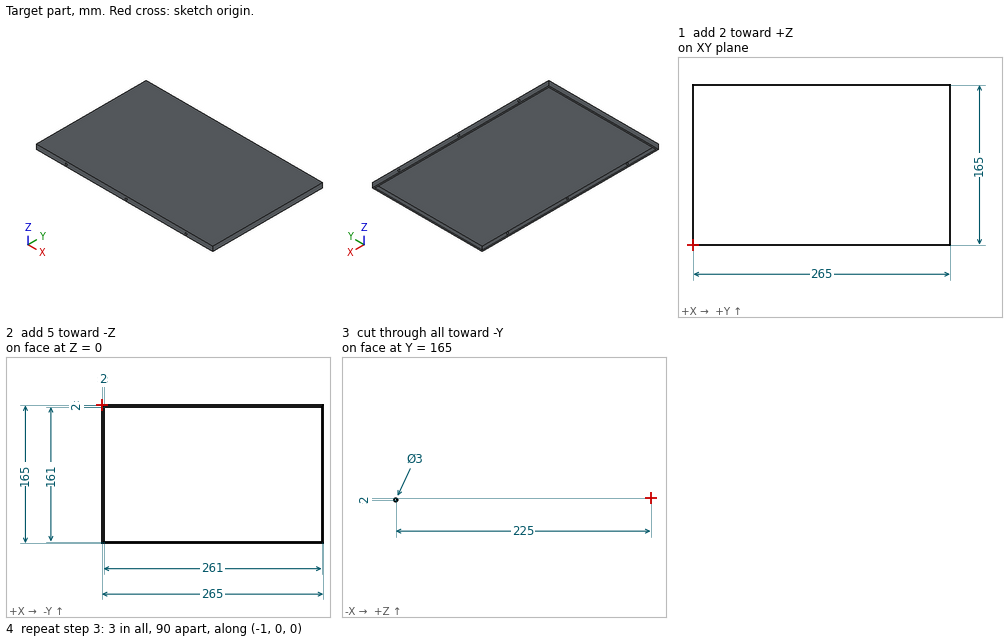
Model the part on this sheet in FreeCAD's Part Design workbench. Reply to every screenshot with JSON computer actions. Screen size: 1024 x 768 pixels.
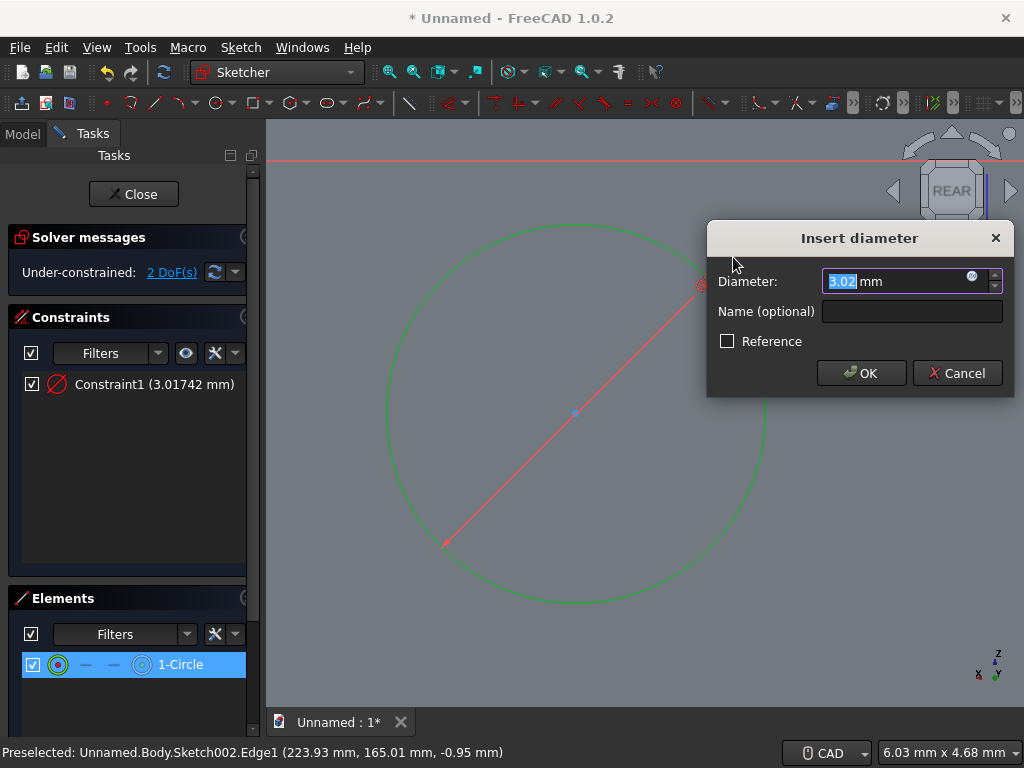
{"action": "type", "text": "3"}
{"action": "key", "text": "Return"}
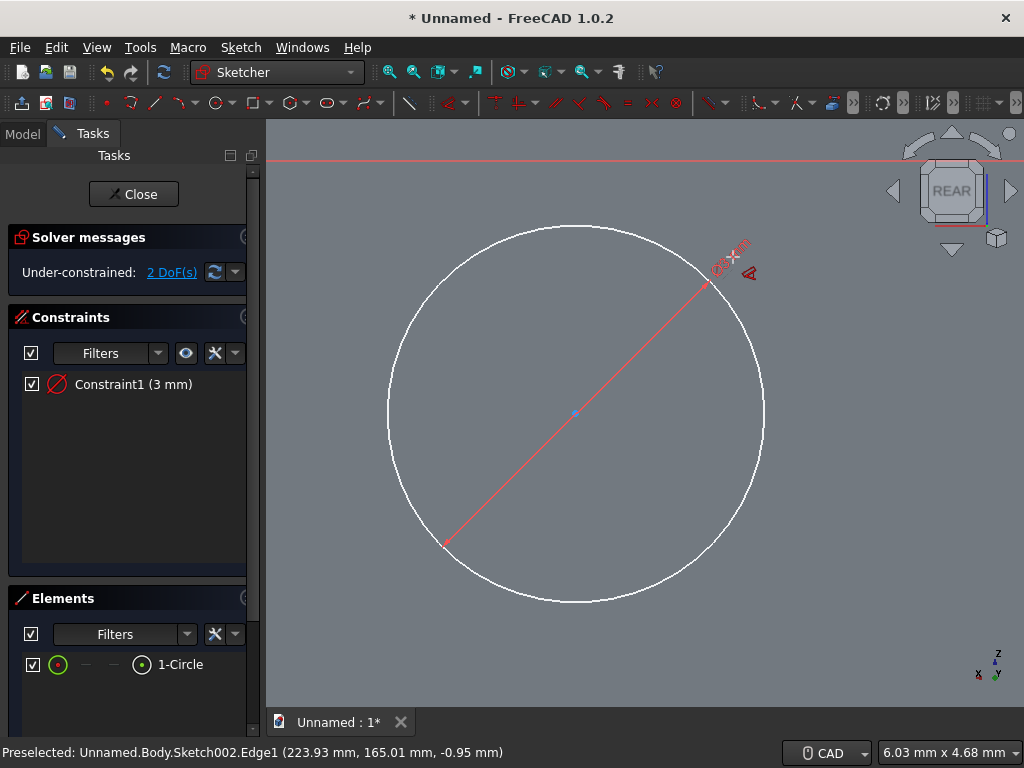
{"action": "left_click", "coordinate": [576, 414]}
{"action": "left_click", "coordinate": [542, 288]}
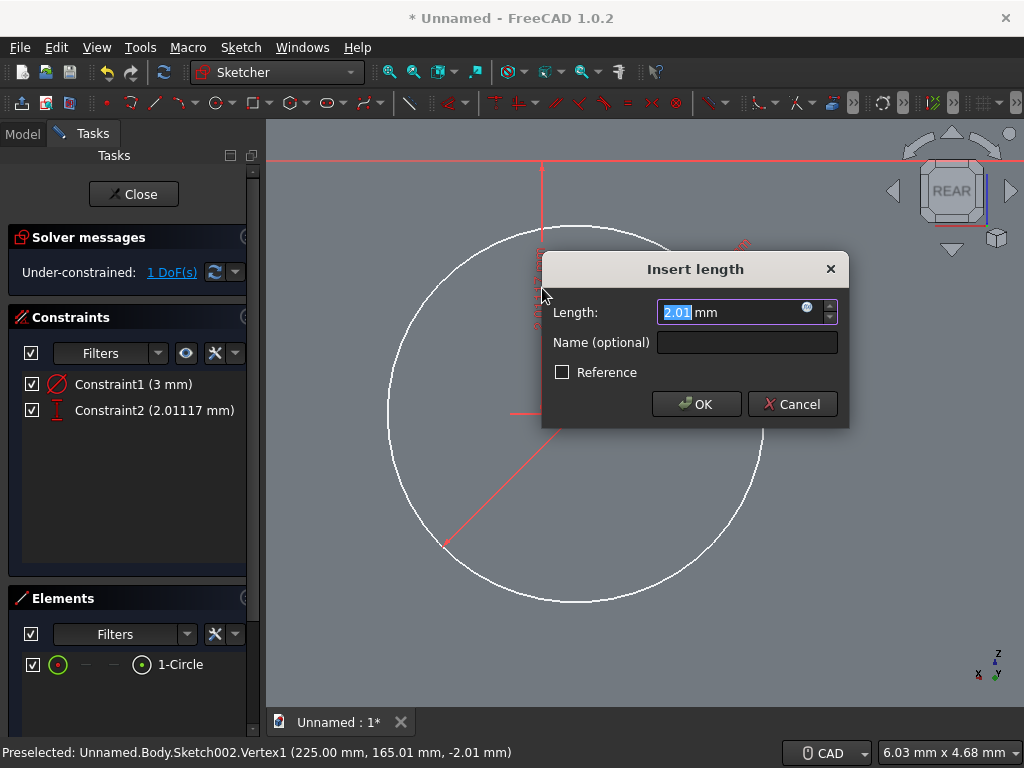
{"action": "type", "text": "2"}
{"action": "key", "text": "Return"}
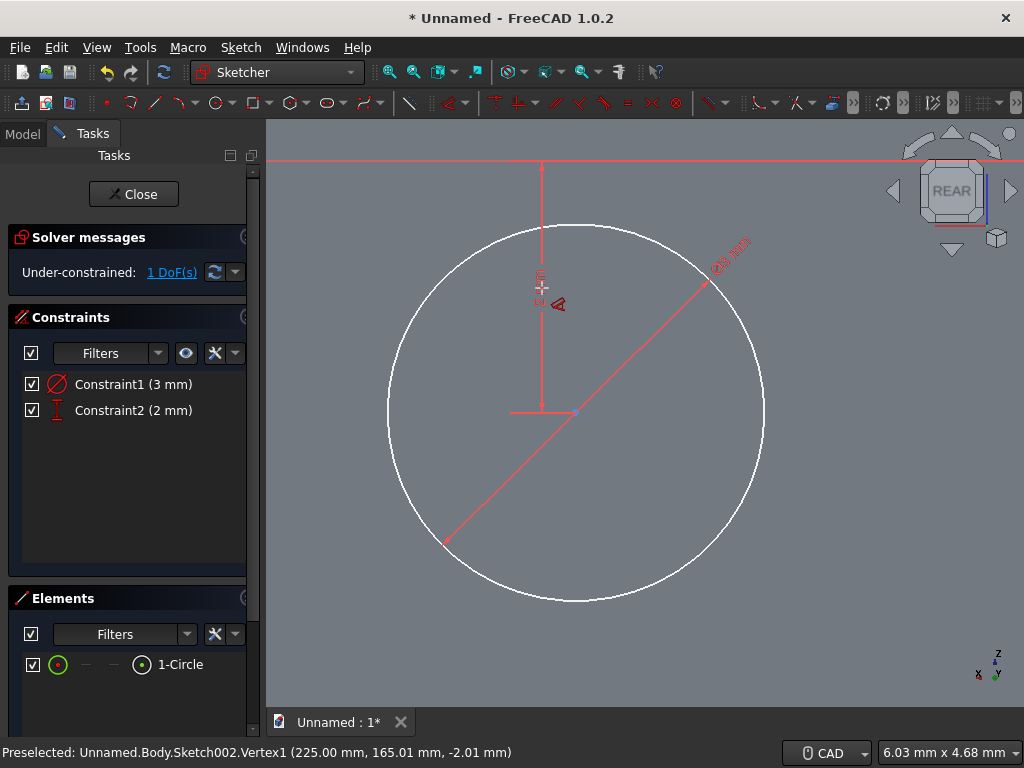
{"action": "left_click", "coordinate": [576, 413]}
{"action": "left_click", "coordinate": [718, 447]}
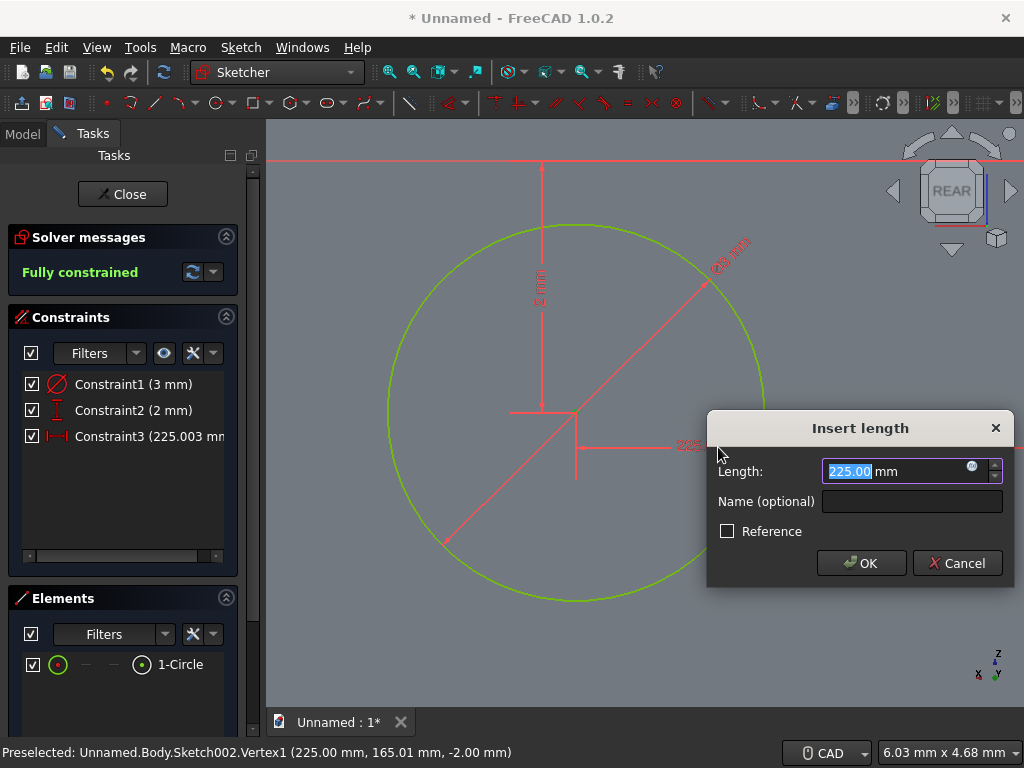
{"action": "type", "text": "225"}
{"action": "key", "text": "Return"}
{"action": "key", "text": "Escape"}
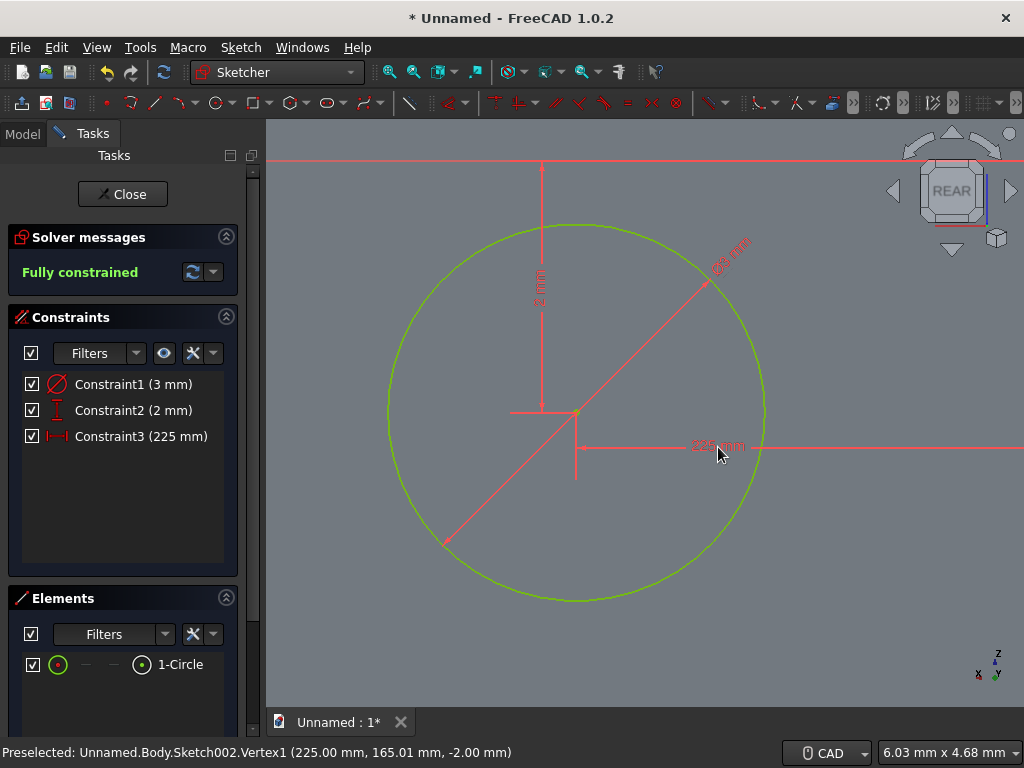
{"action": "left_click", "coordinate": [123, 194]}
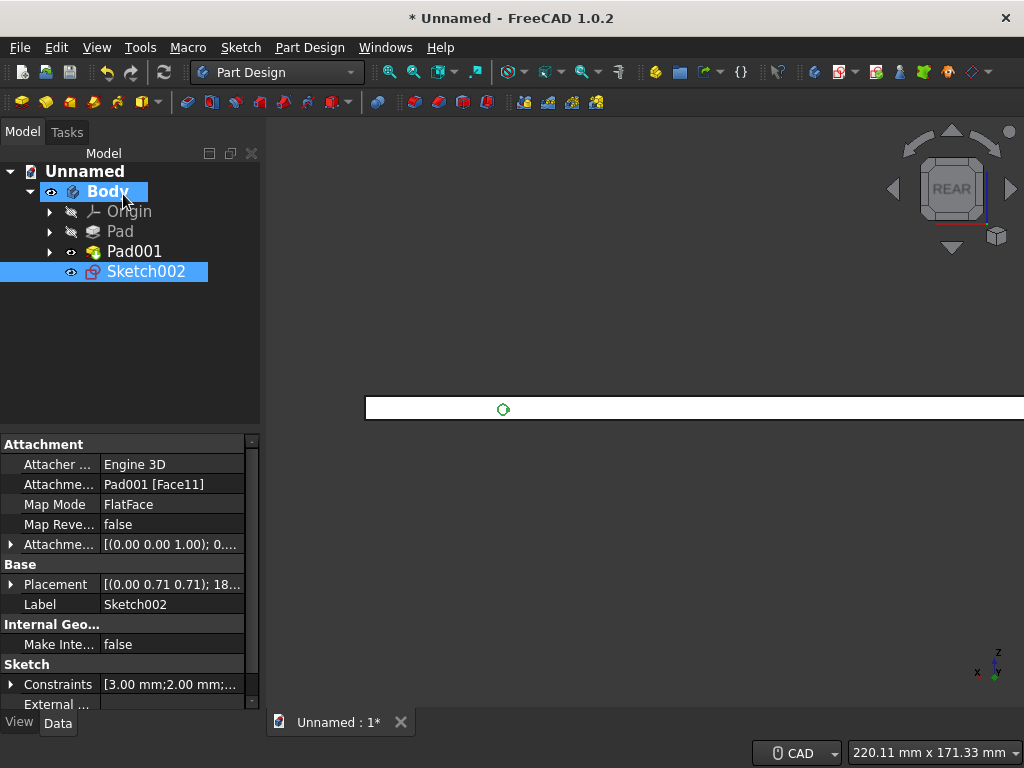
{"action": "left_click", "coordinate": [188, 102]}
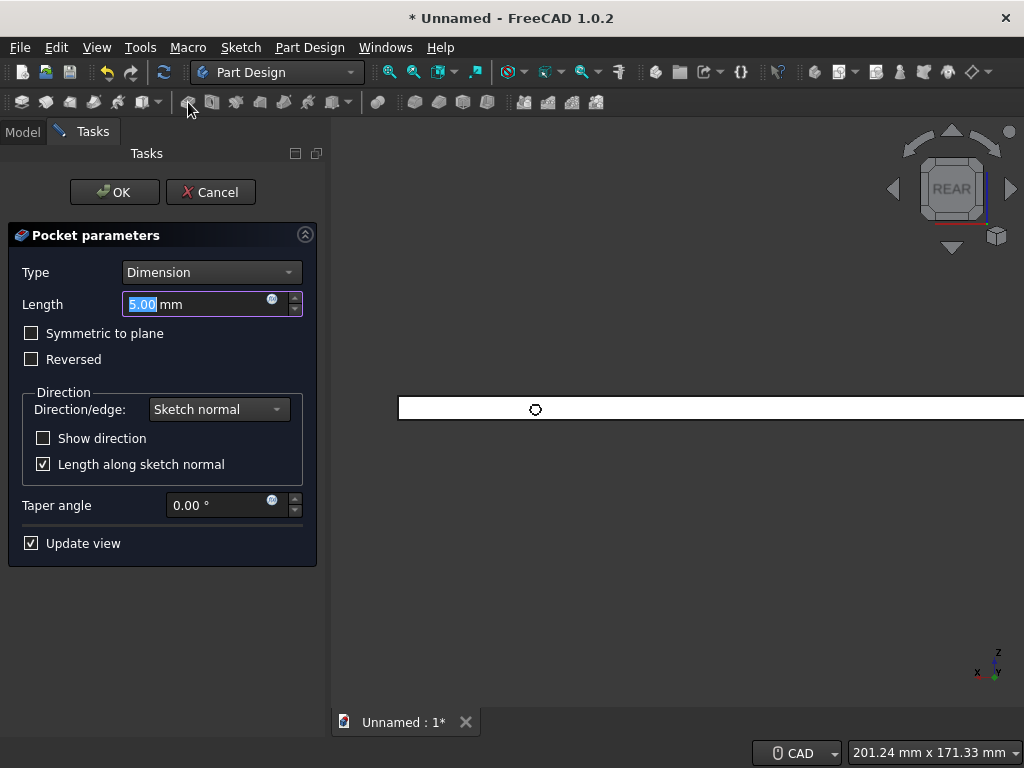
{"action": "left_click", "coordinate": [212, 272]}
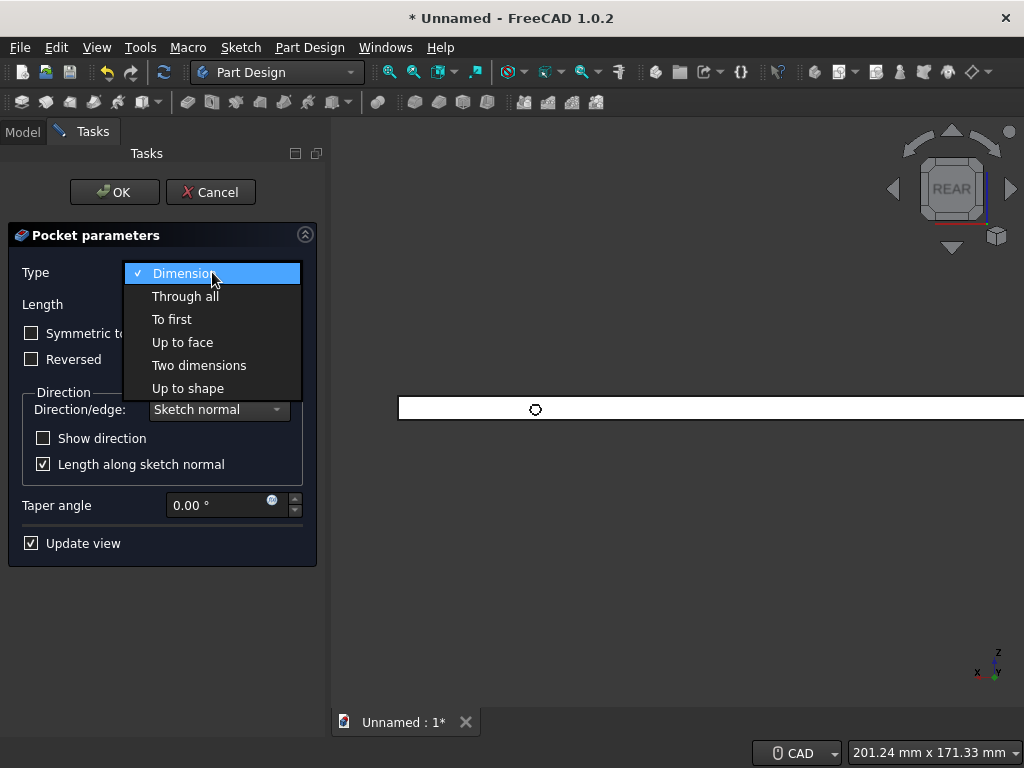
{"action": "left_click", "coordinate": [212, 296]}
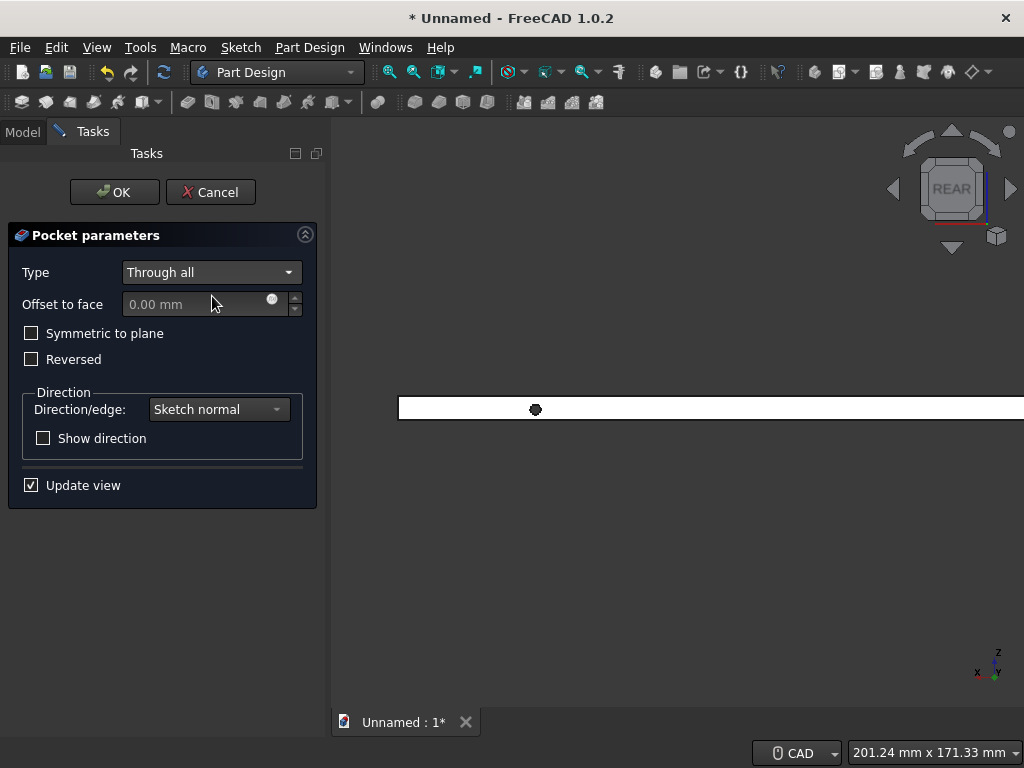
{"action": "left_click", "coordinate": [115, 192]}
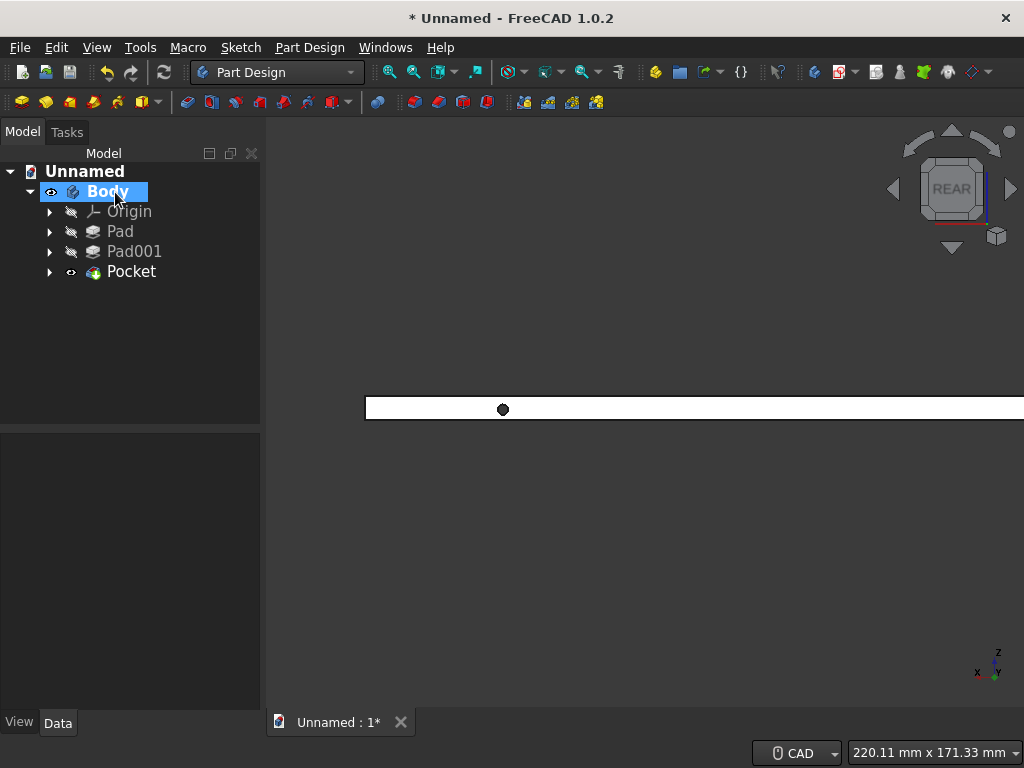
{"action": "key", "text": "v f"}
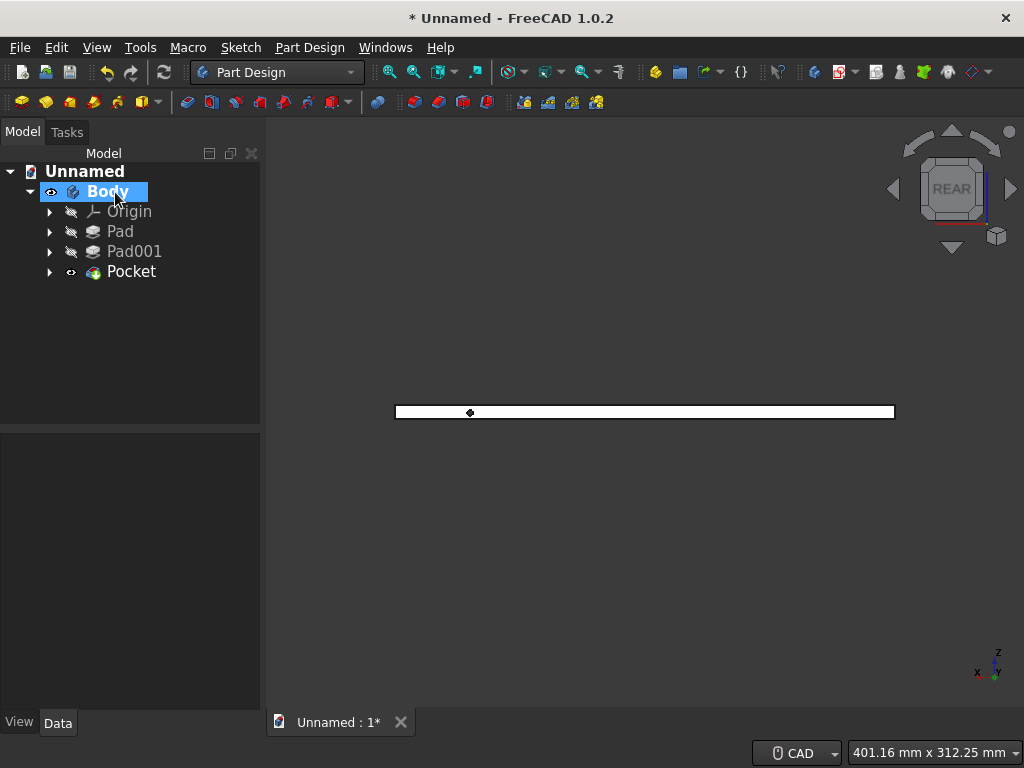
{"action": "left_click", "coordinate": [116, 272]}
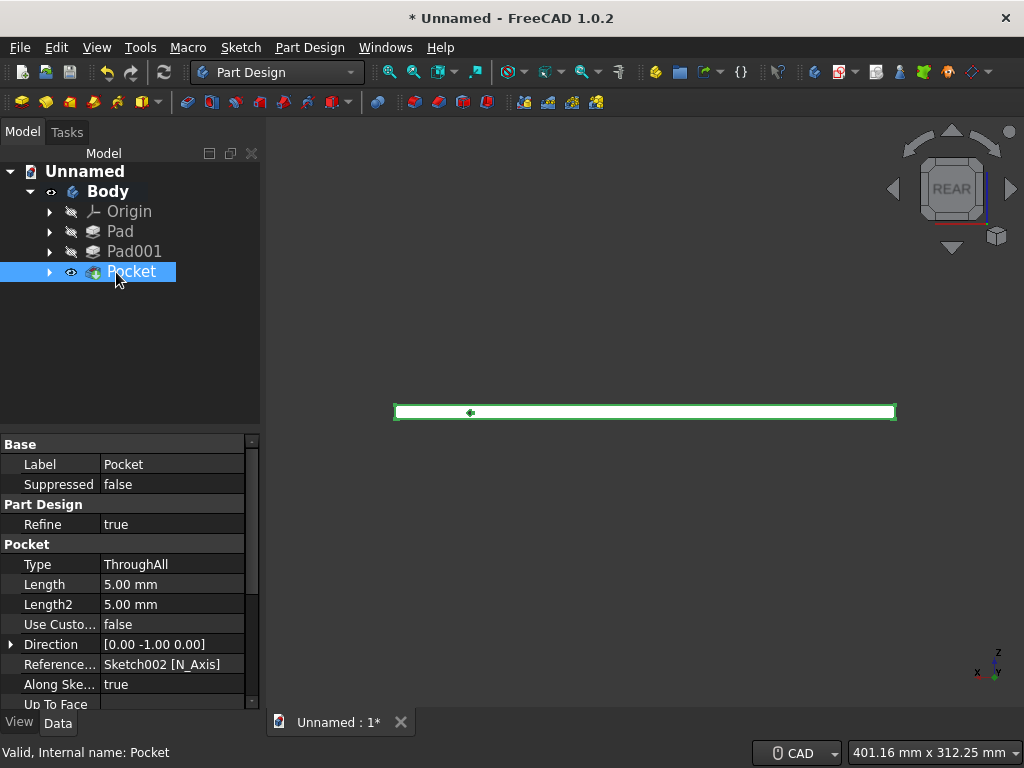
{"action": "left_click", "coordinate": [548, 102]}